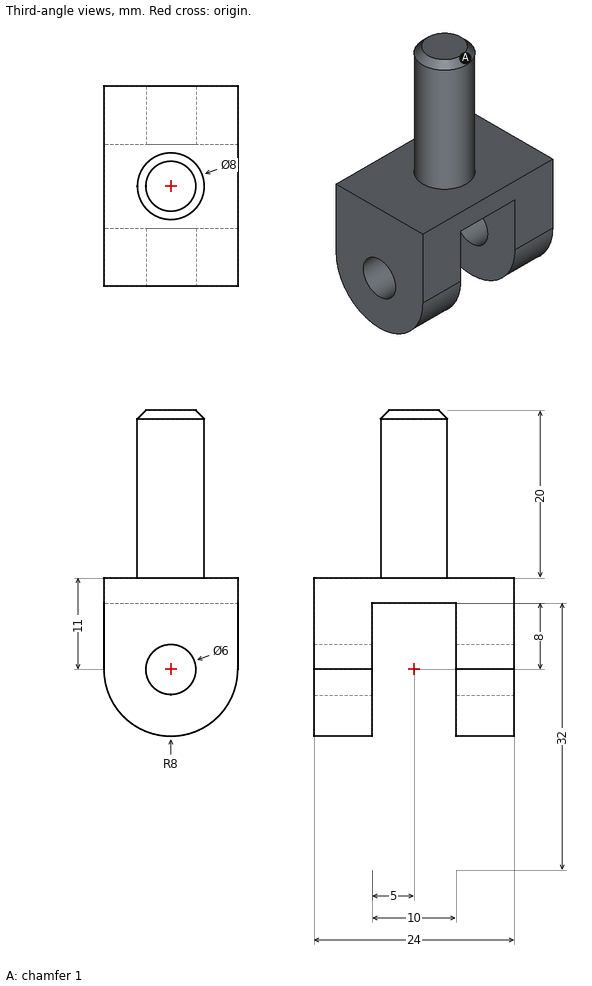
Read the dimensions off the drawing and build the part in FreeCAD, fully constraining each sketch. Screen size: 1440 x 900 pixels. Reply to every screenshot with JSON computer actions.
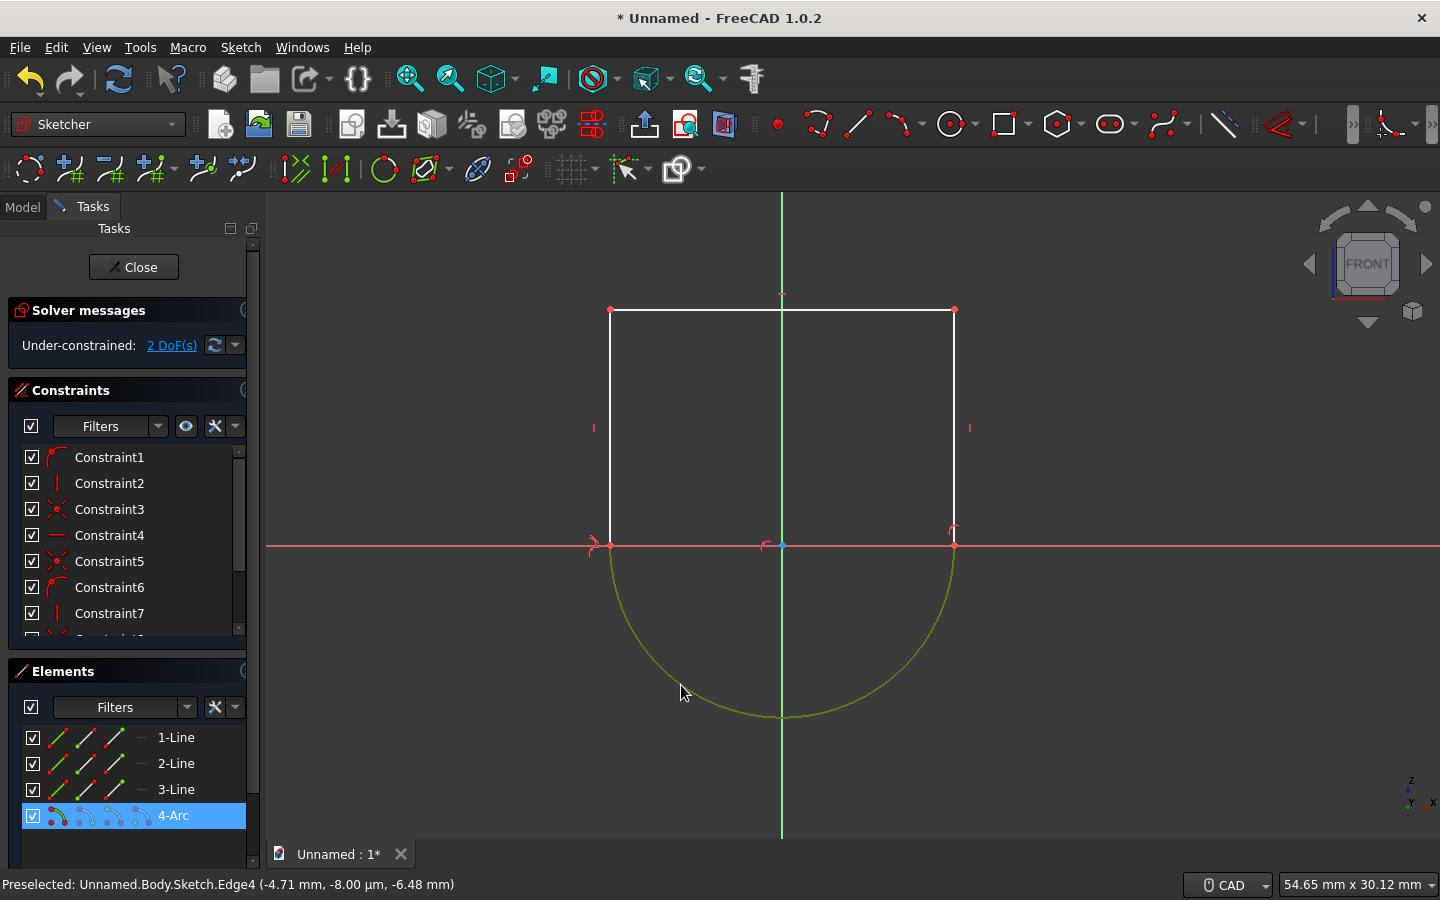
{"action": "left_click", "coordinate": [1304, 124]}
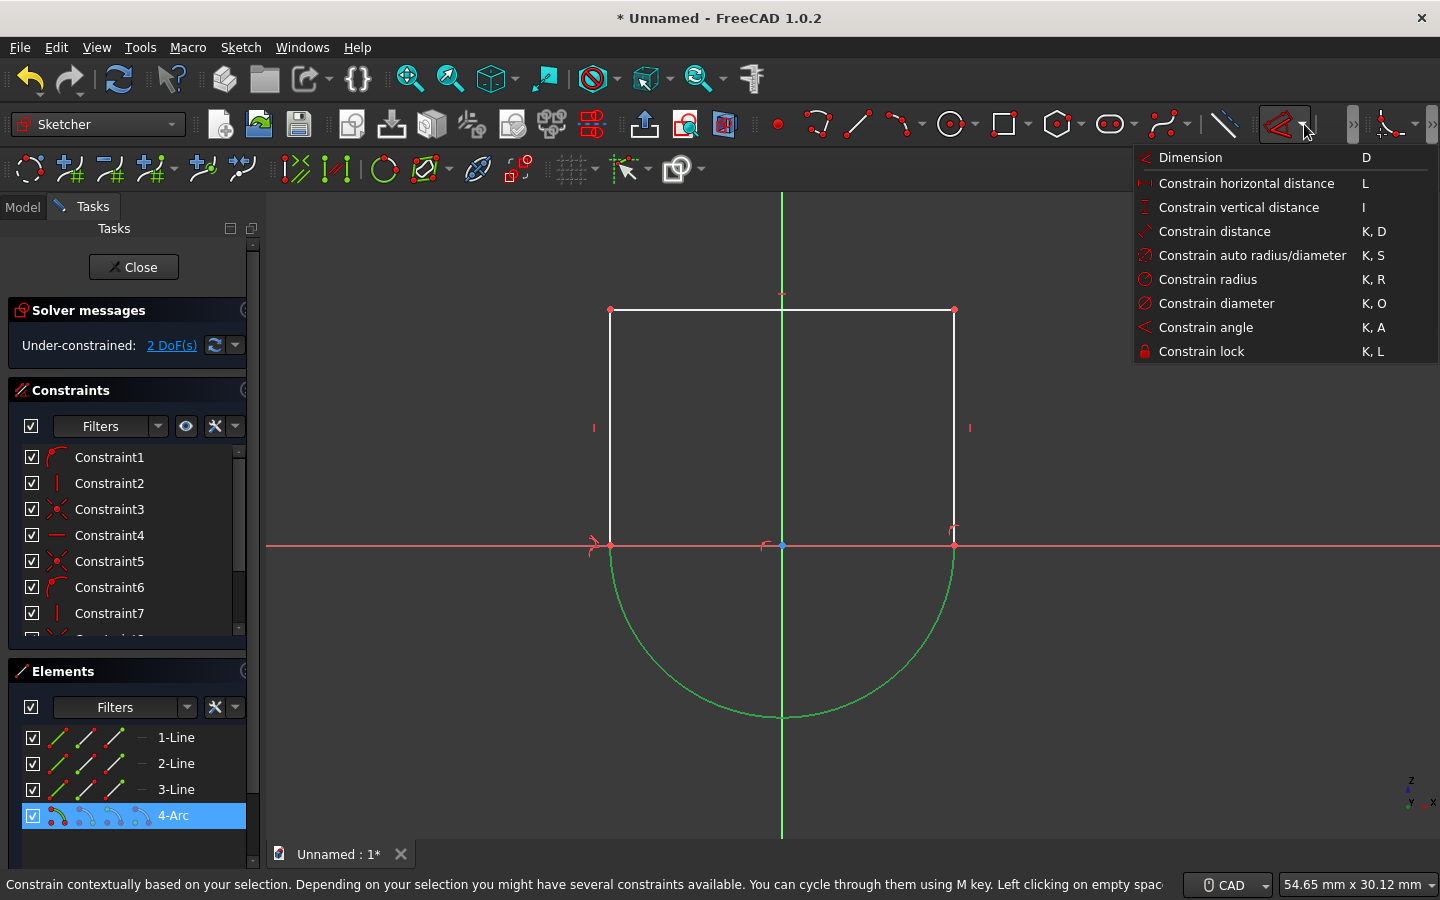
{"action": "left_click", "coordinate": [1286, 279]}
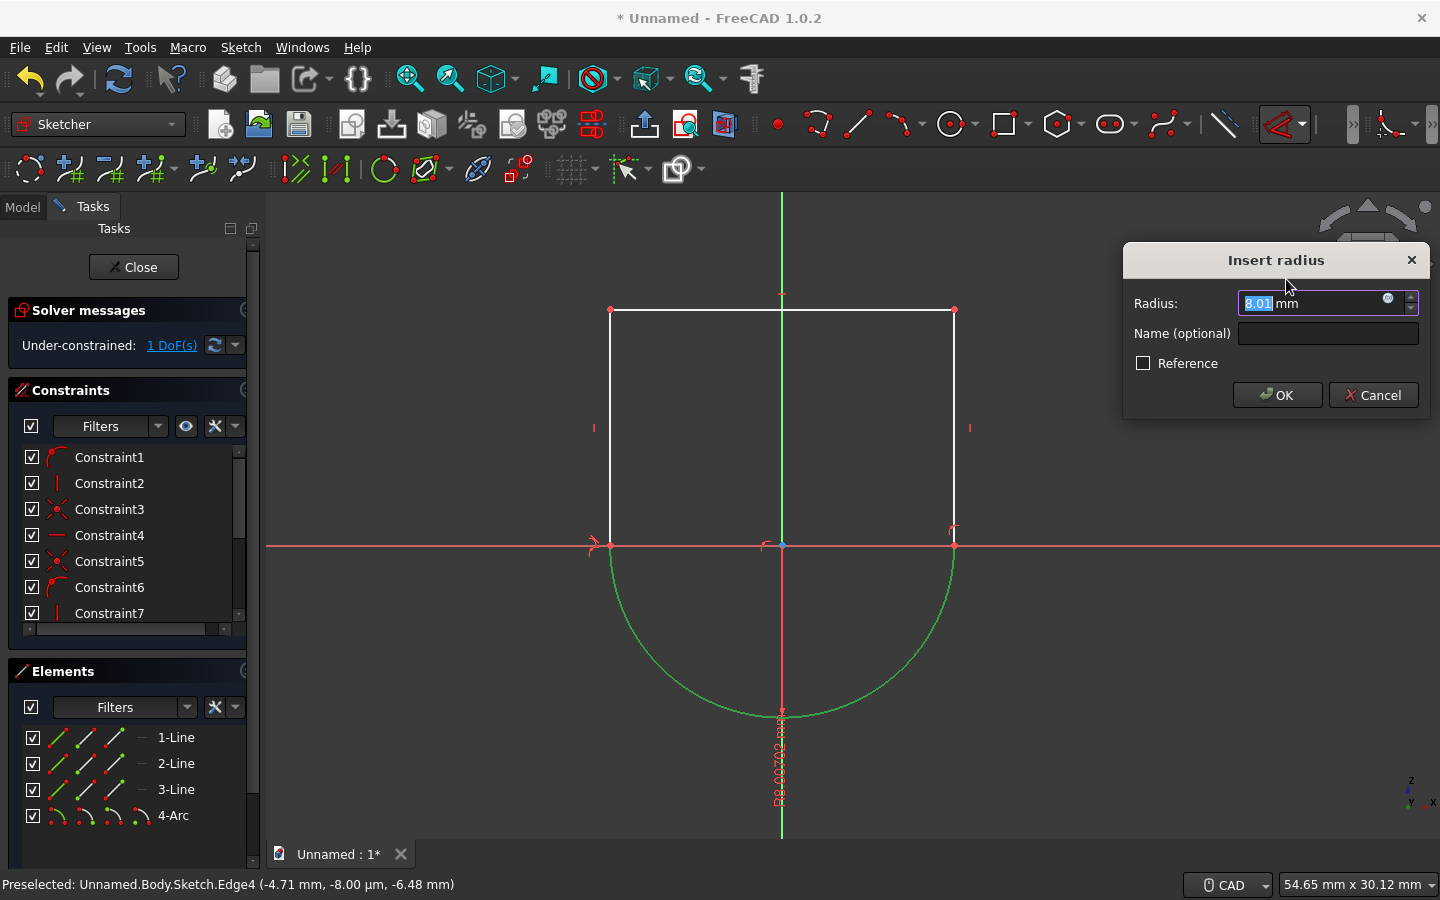
{"action": "type", "text": "8"}
{"action": "key", "text": "Return"}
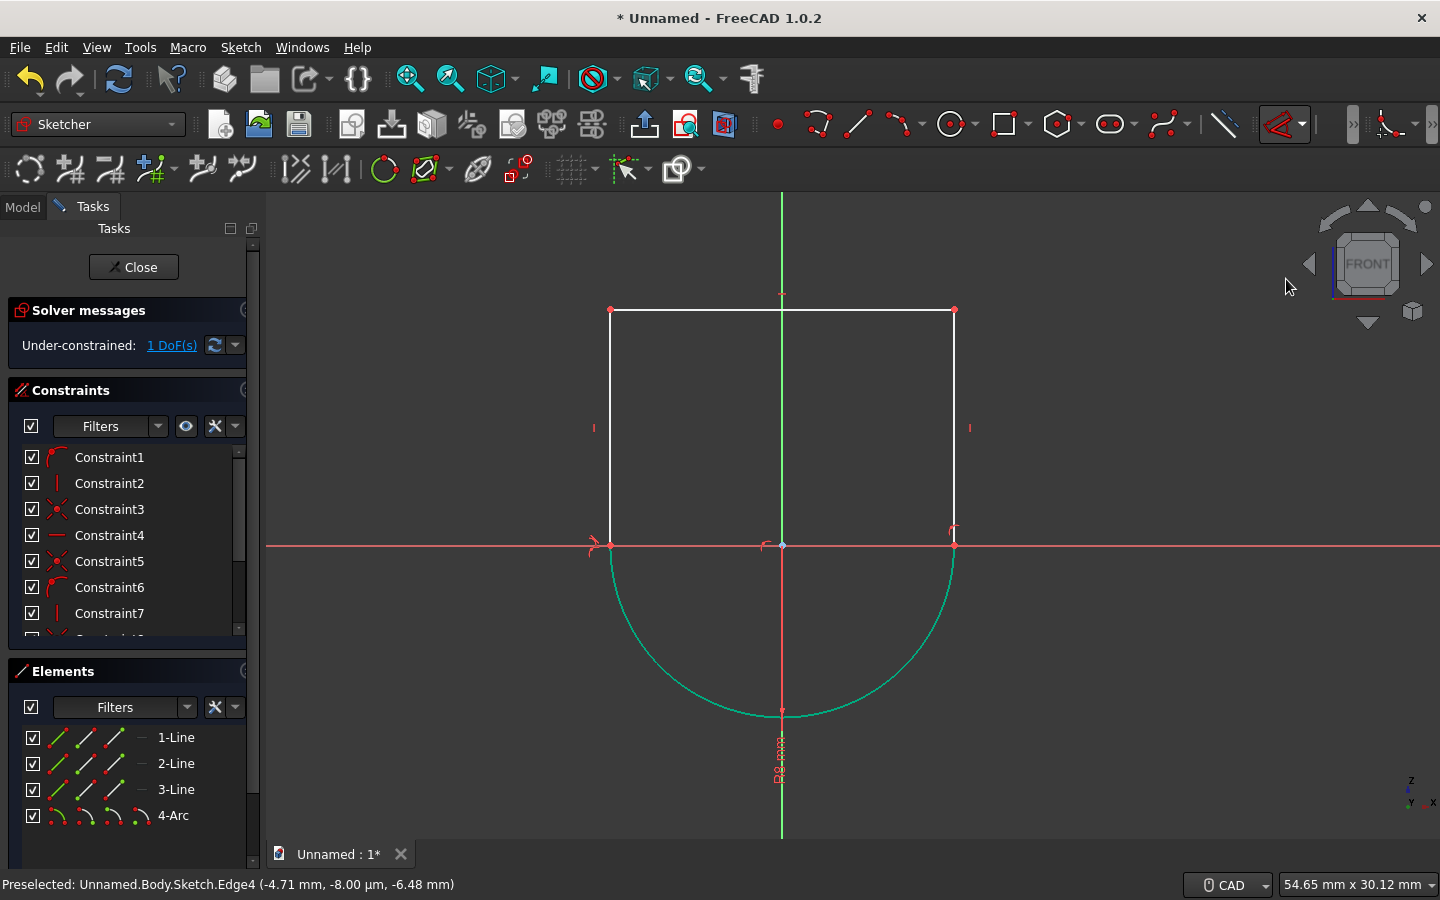
{"action": "left_click", "coordinate": [610, 475]}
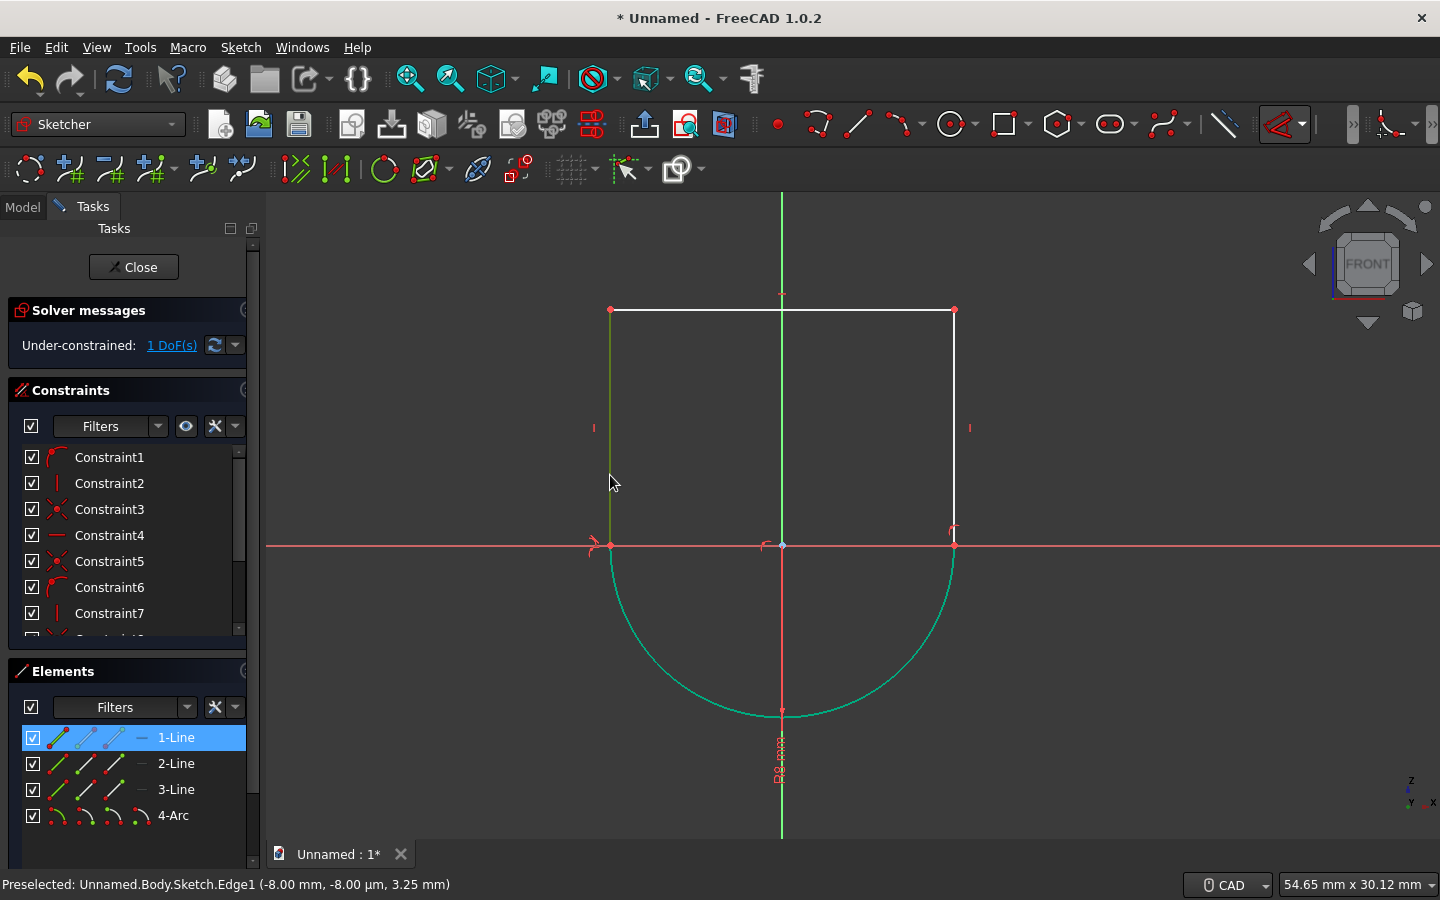
{"action": "left_click", "coordinate": [1304, 124]}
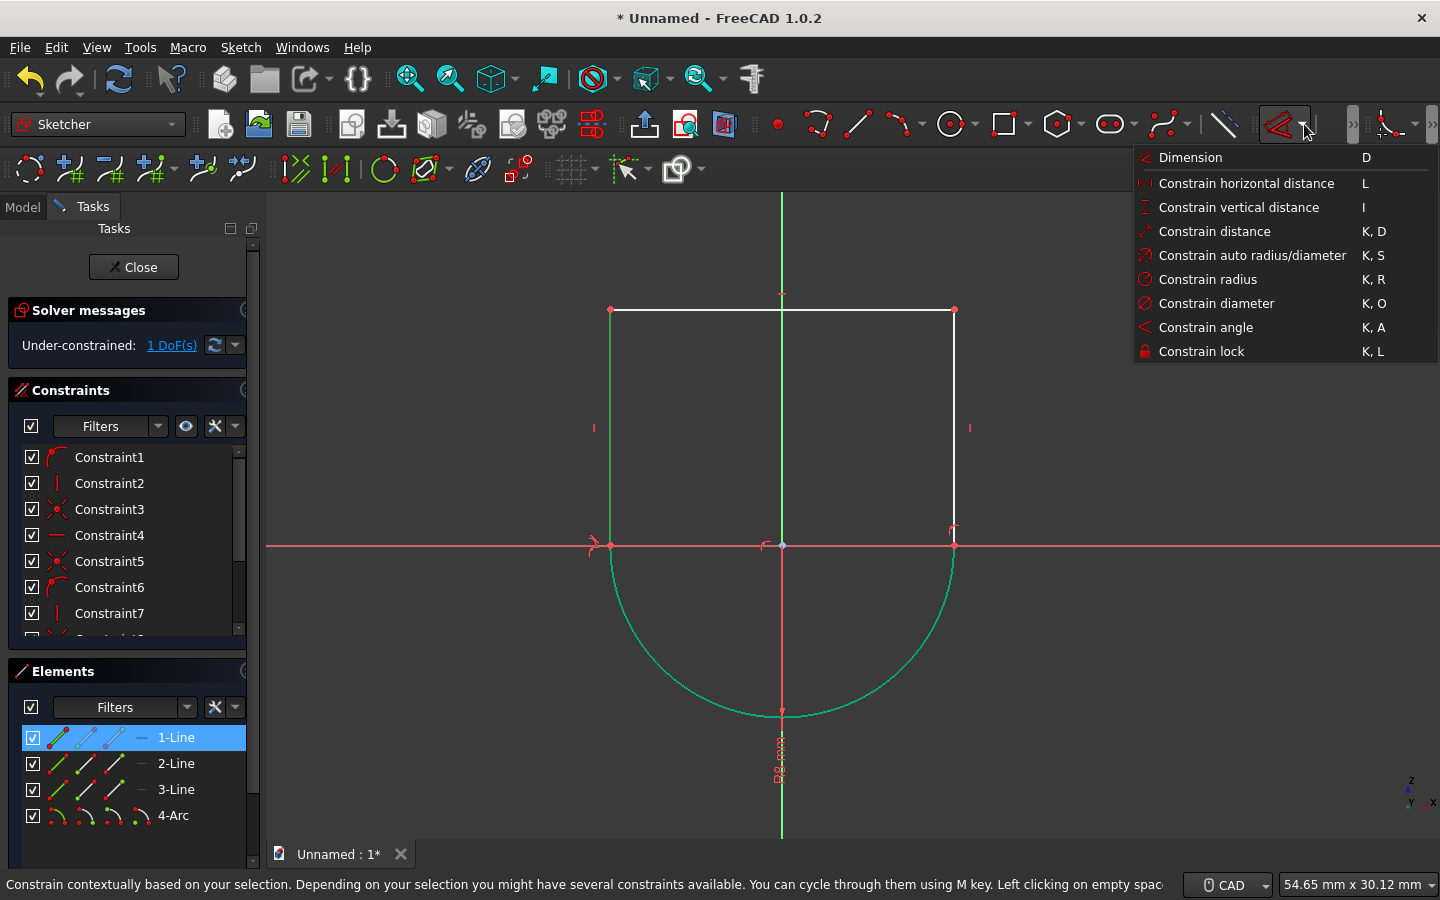
{"action": "left_click", "coordinate": [1286, 207]}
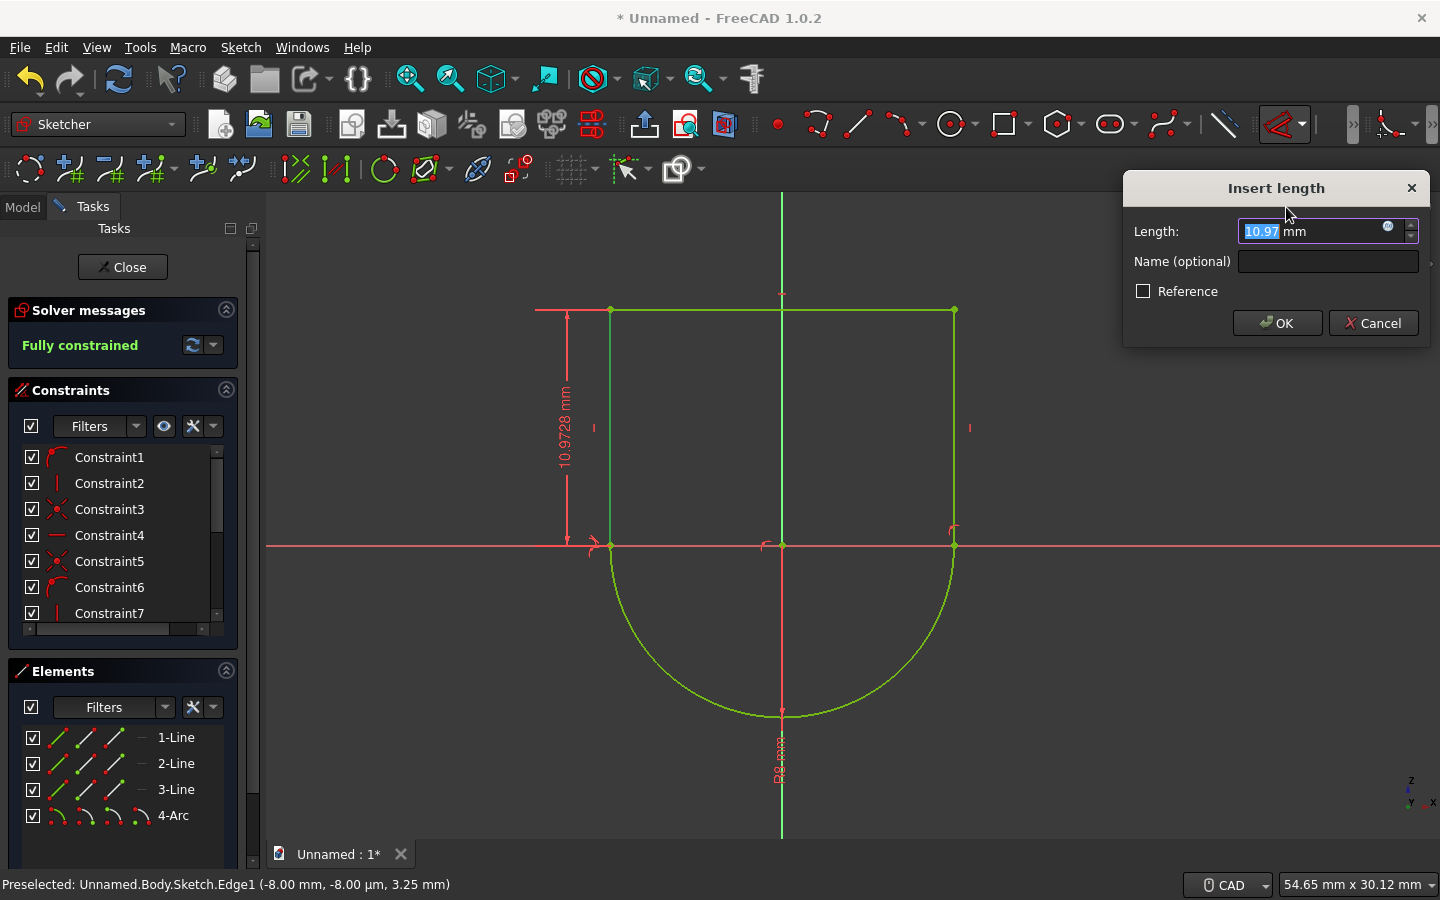
{"action": "type", "text": "11"}
{"action": "key", "text": "Return"}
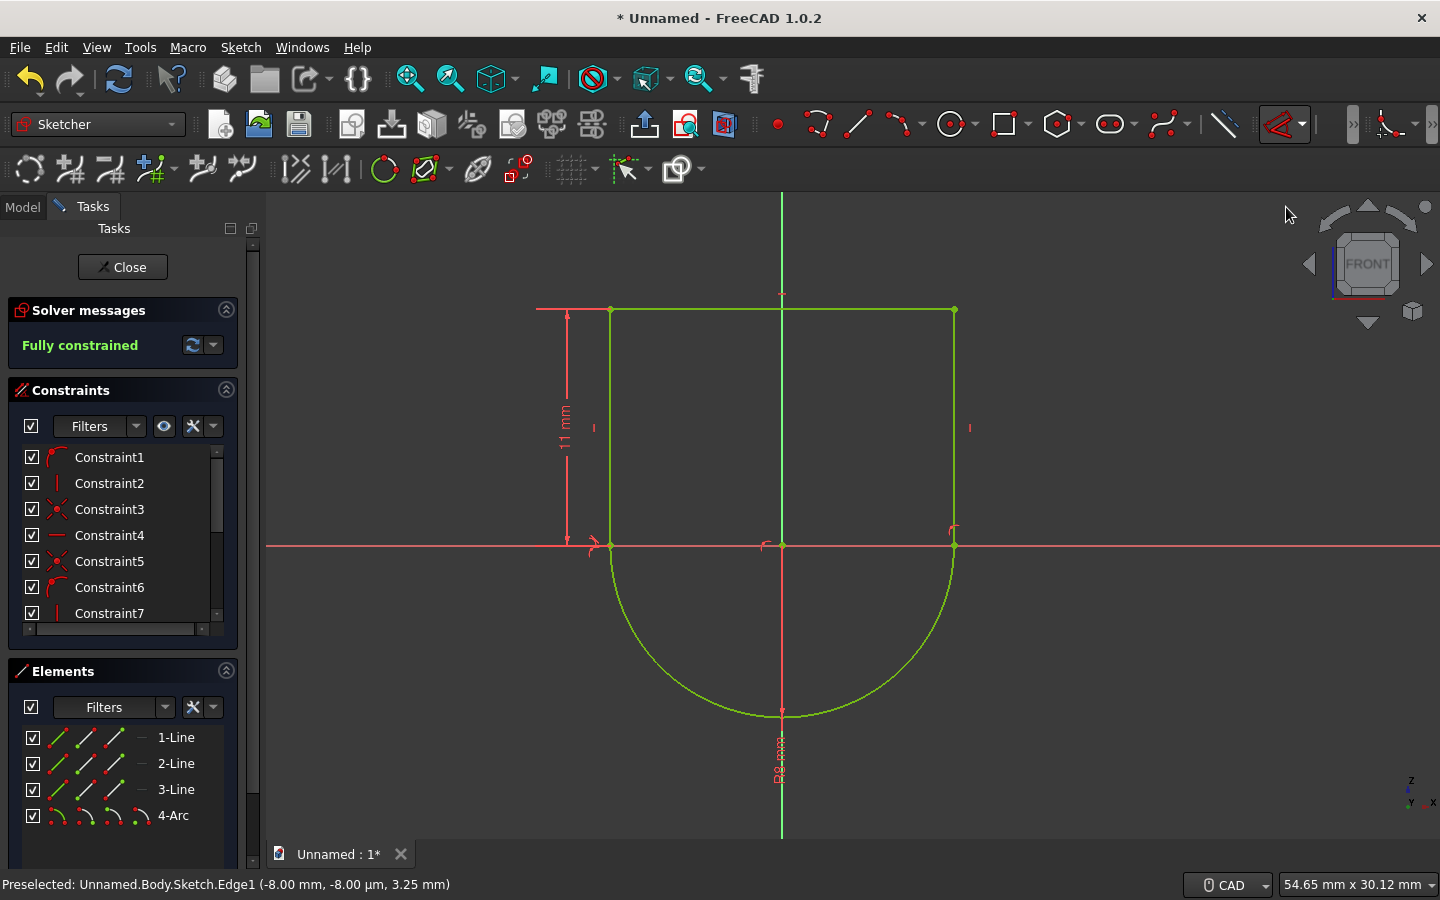
{"action": "left_click", "coordinate": [123, 267]}